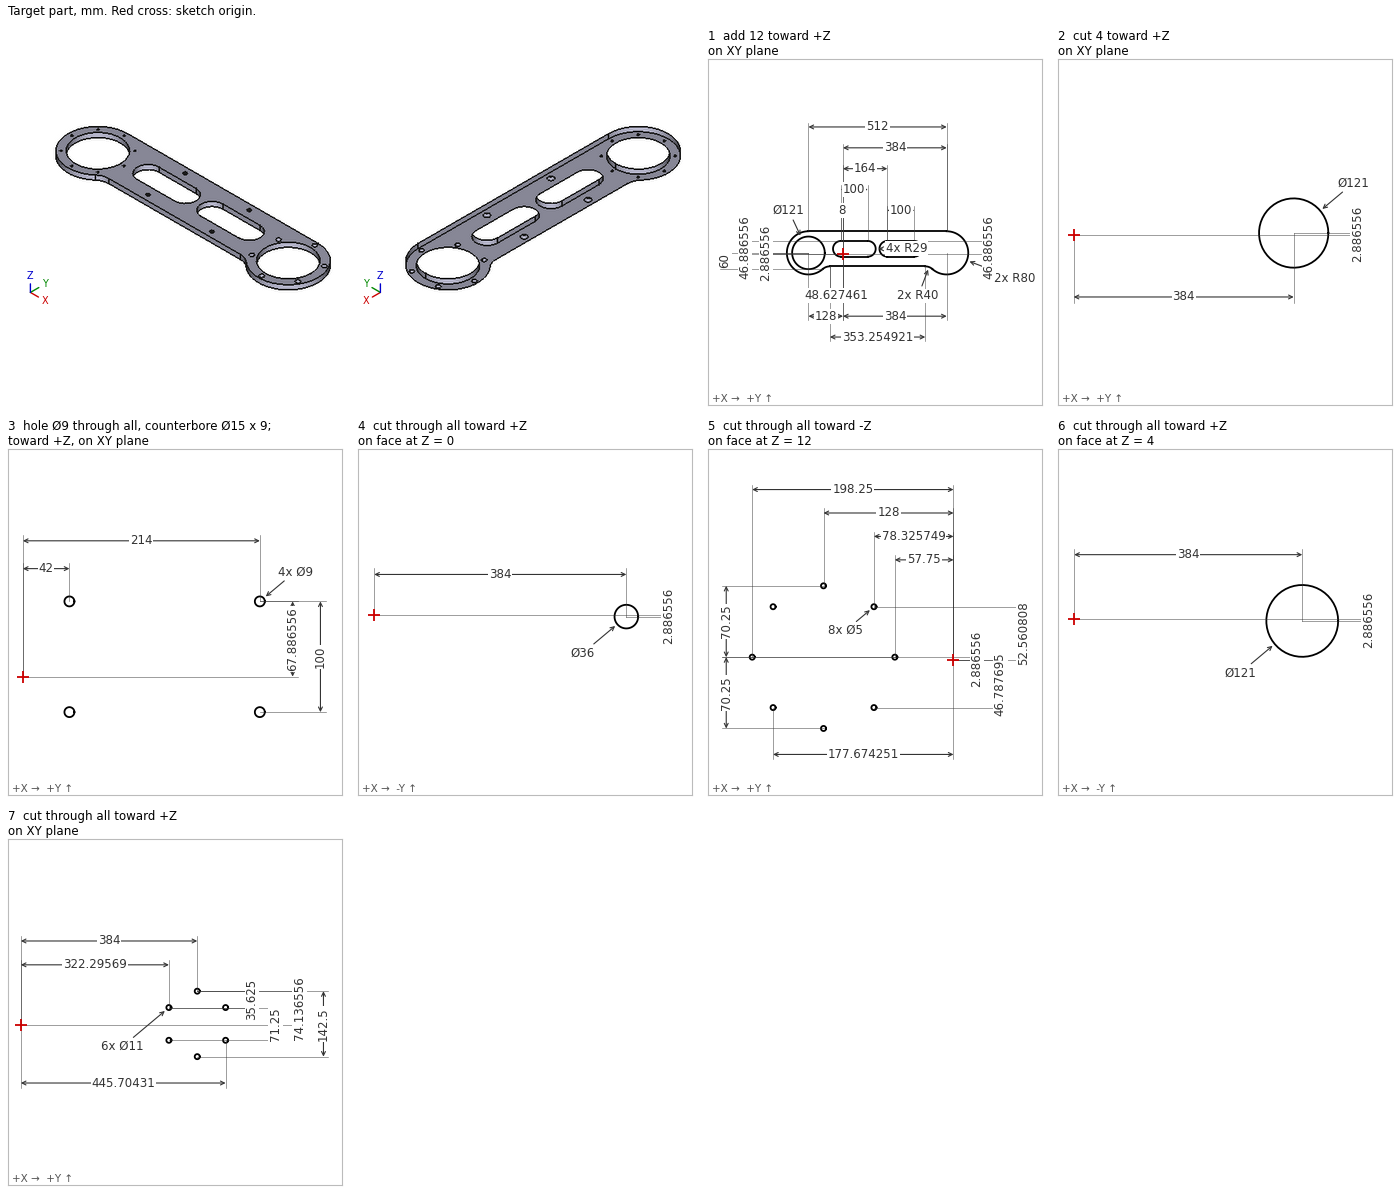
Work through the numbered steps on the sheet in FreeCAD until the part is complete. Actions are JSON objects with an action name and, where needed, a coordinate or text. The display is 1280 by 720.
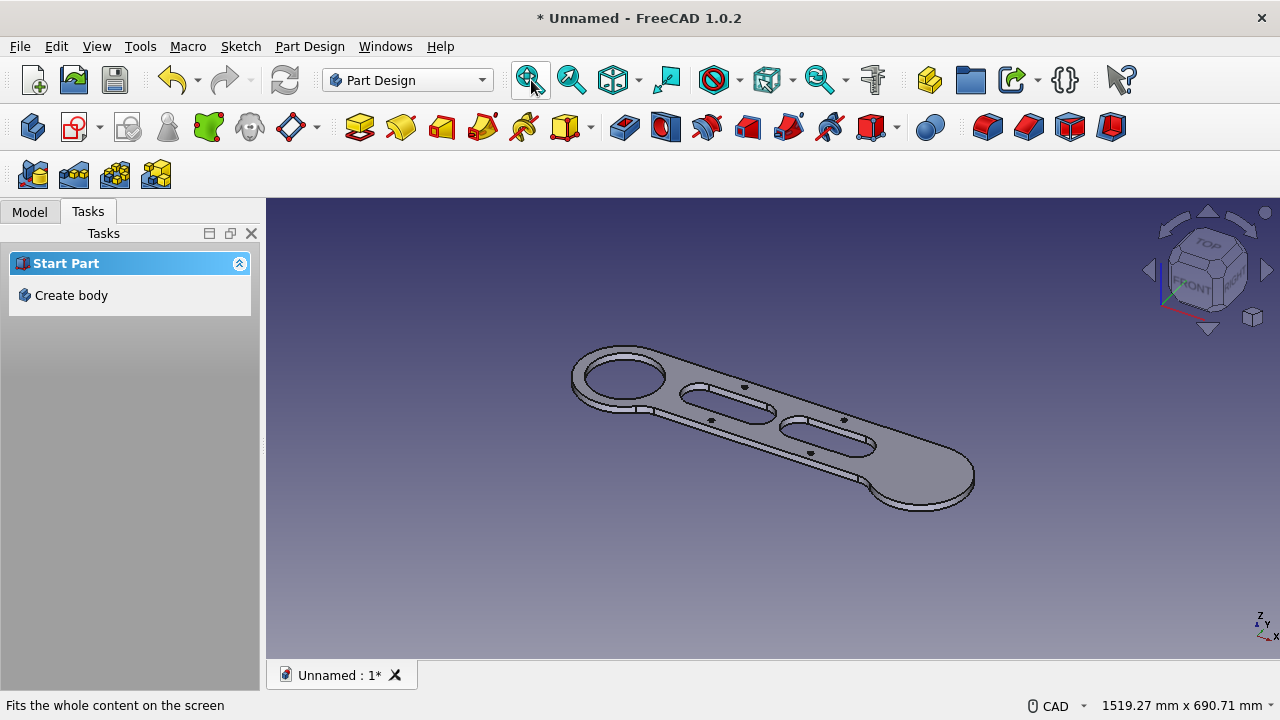
{"action": "key", "text": "5"}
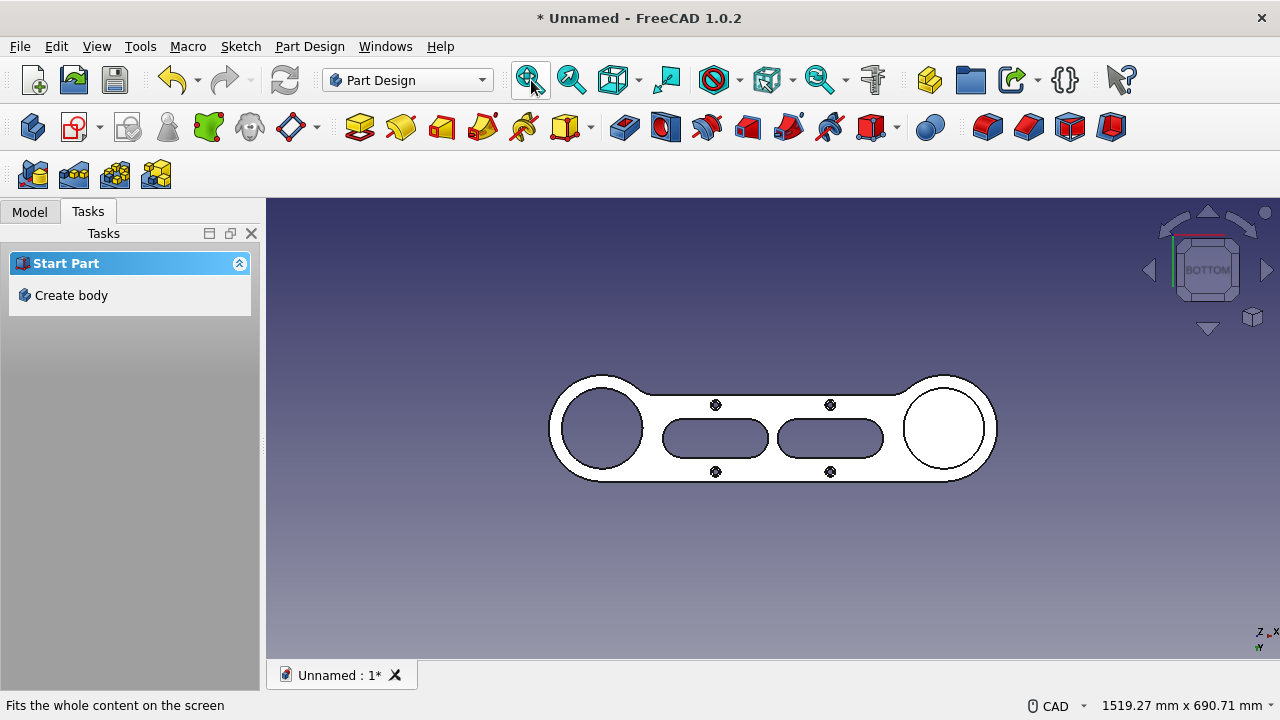
{"action": "left_click", "coordinate": [531, 80]}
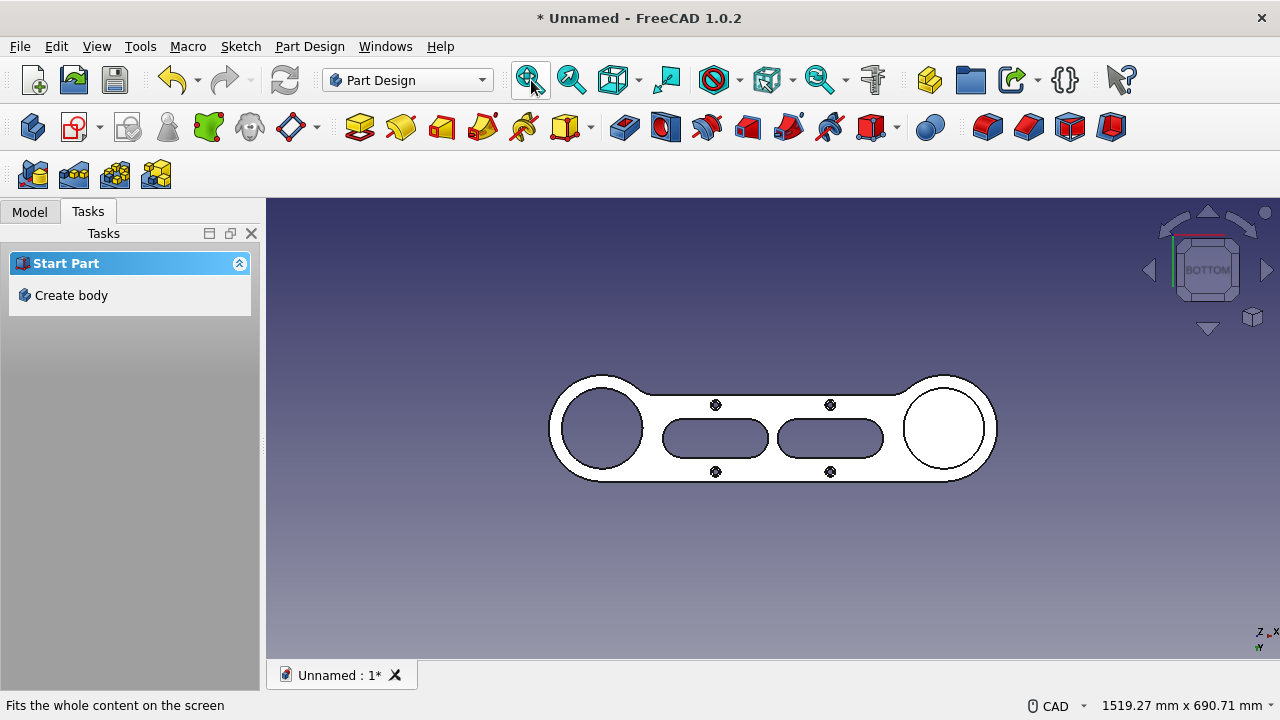
{"action": "left_click", "coordinate": [773, 412]}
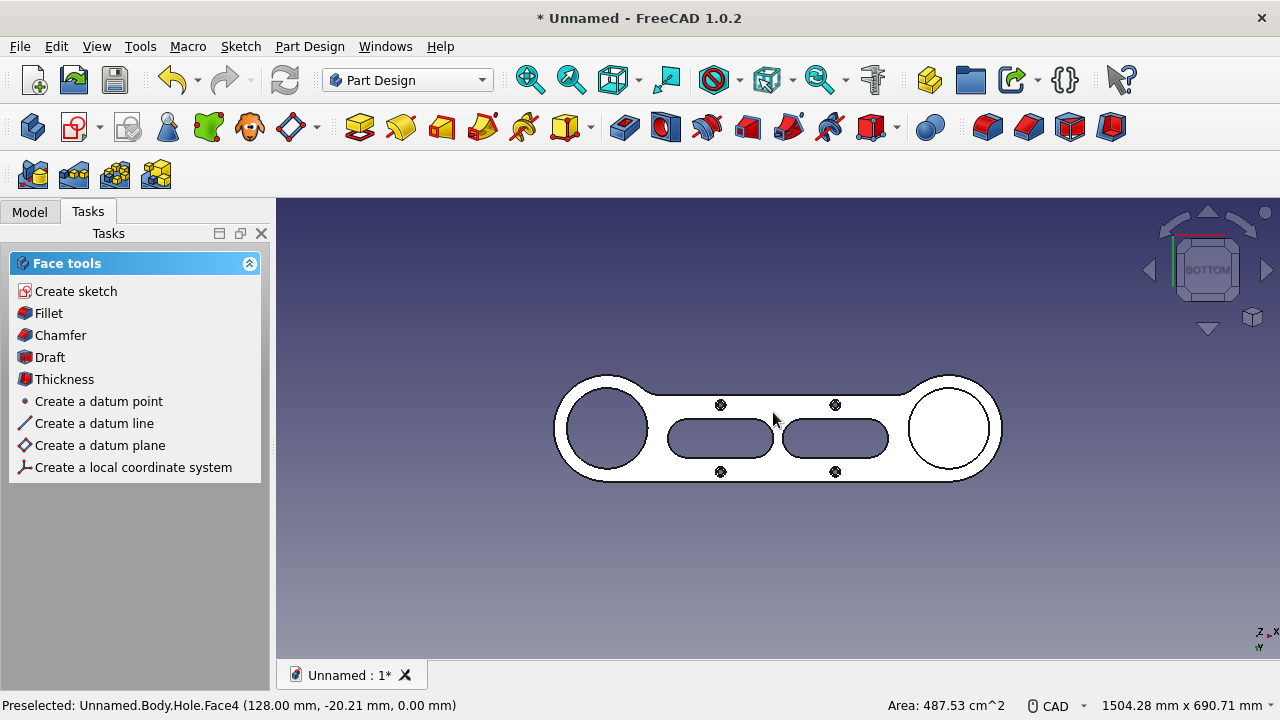
{"action": "left_click", "coordinate": [74, 128]}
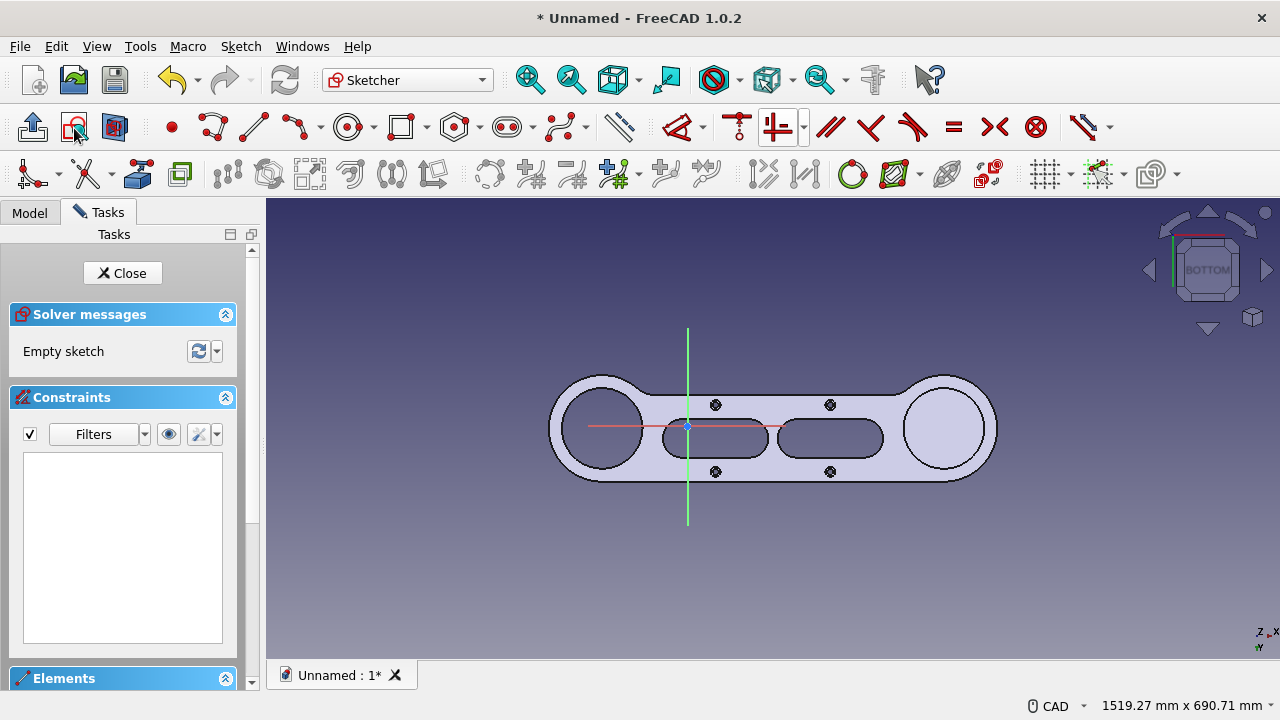
{"action": "scroll", "coordinate": [968, 428], "scroll_direction": "up", "scroll_amount": 12}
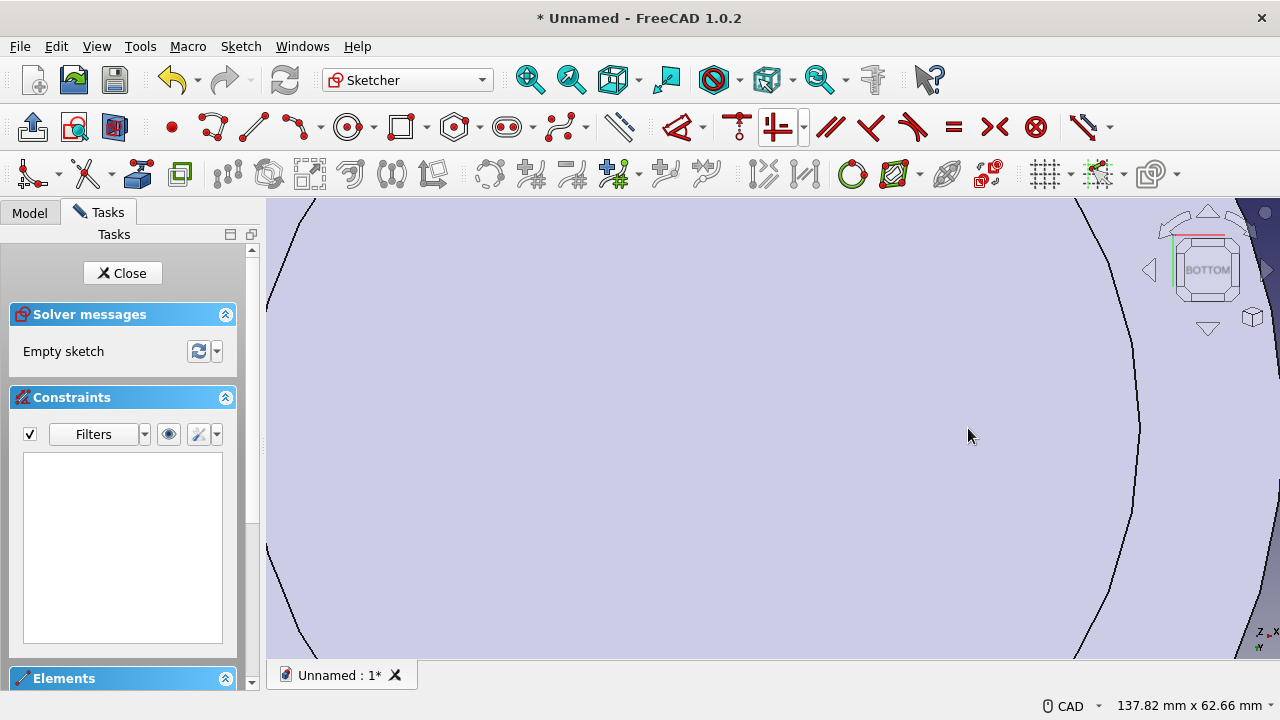
{"action": "left_click", "coordinate": [348, 128]}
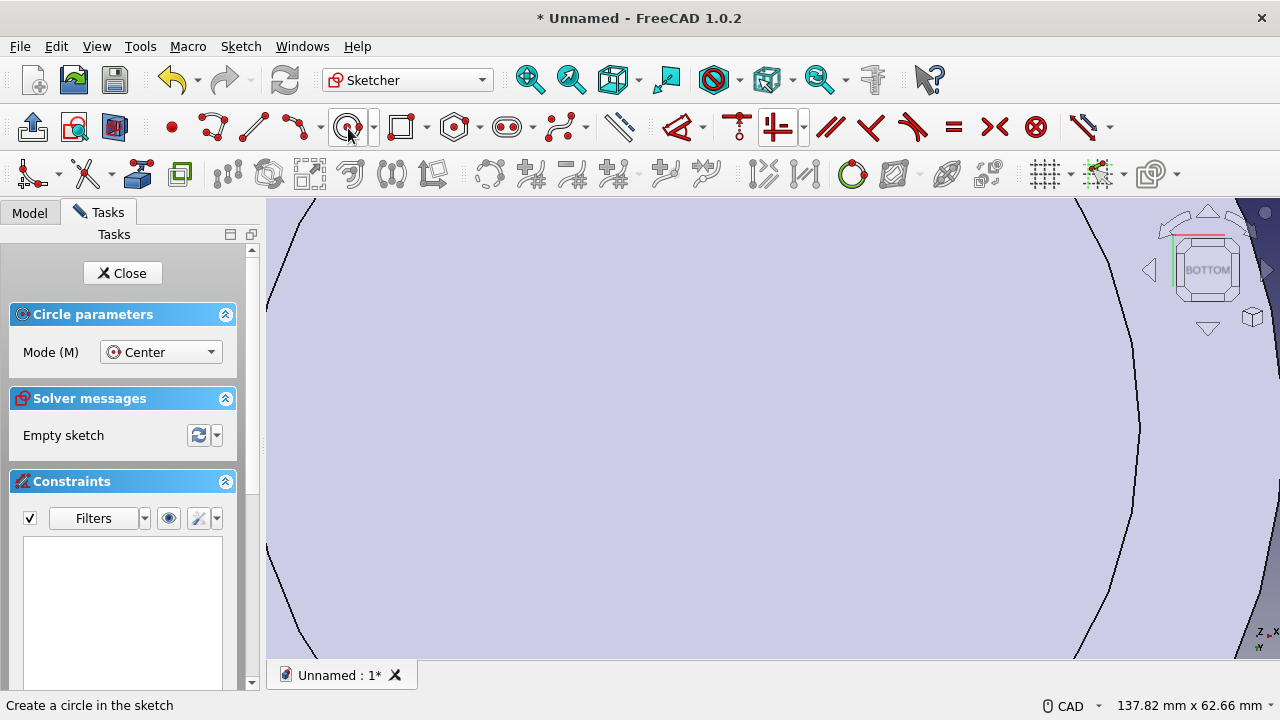
{"action": "left_click", "coordinate": [695, 428]}
{"action": "left_click", "coordinate": [789, 334]}
{"action": "key", "text": "Escape"}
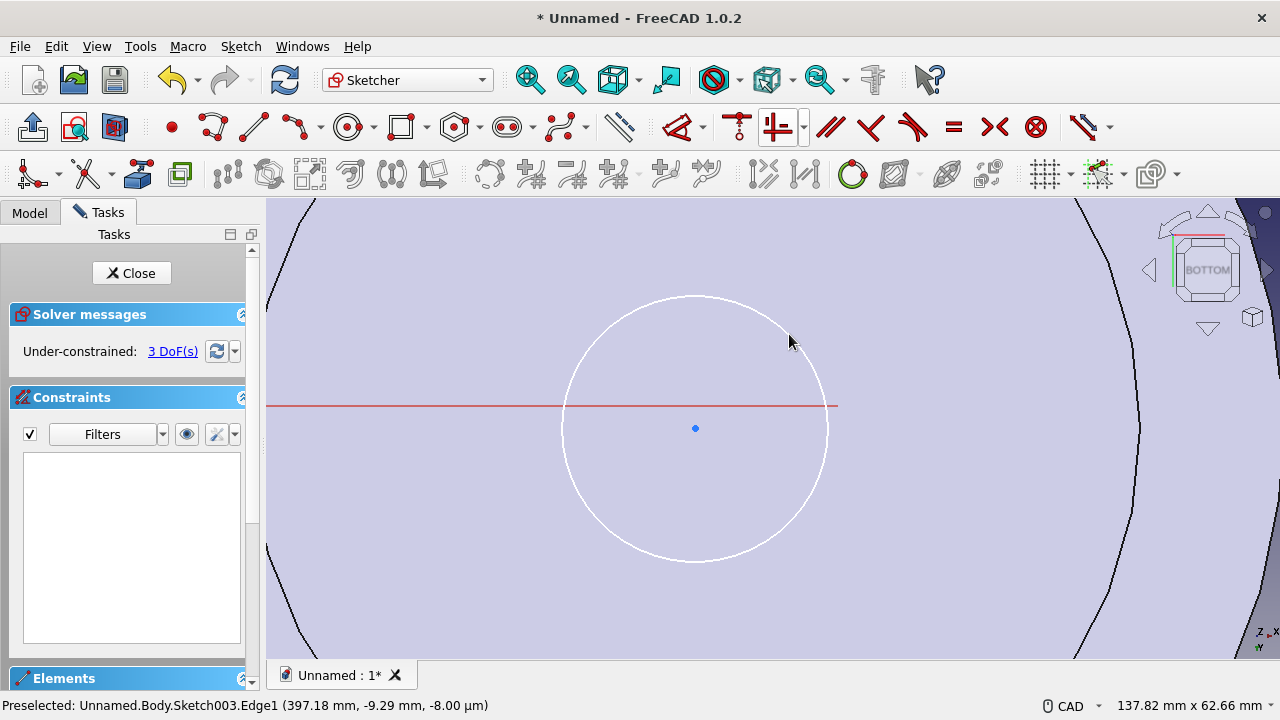
{"action": "left_click", "coordinate": [676, 128]}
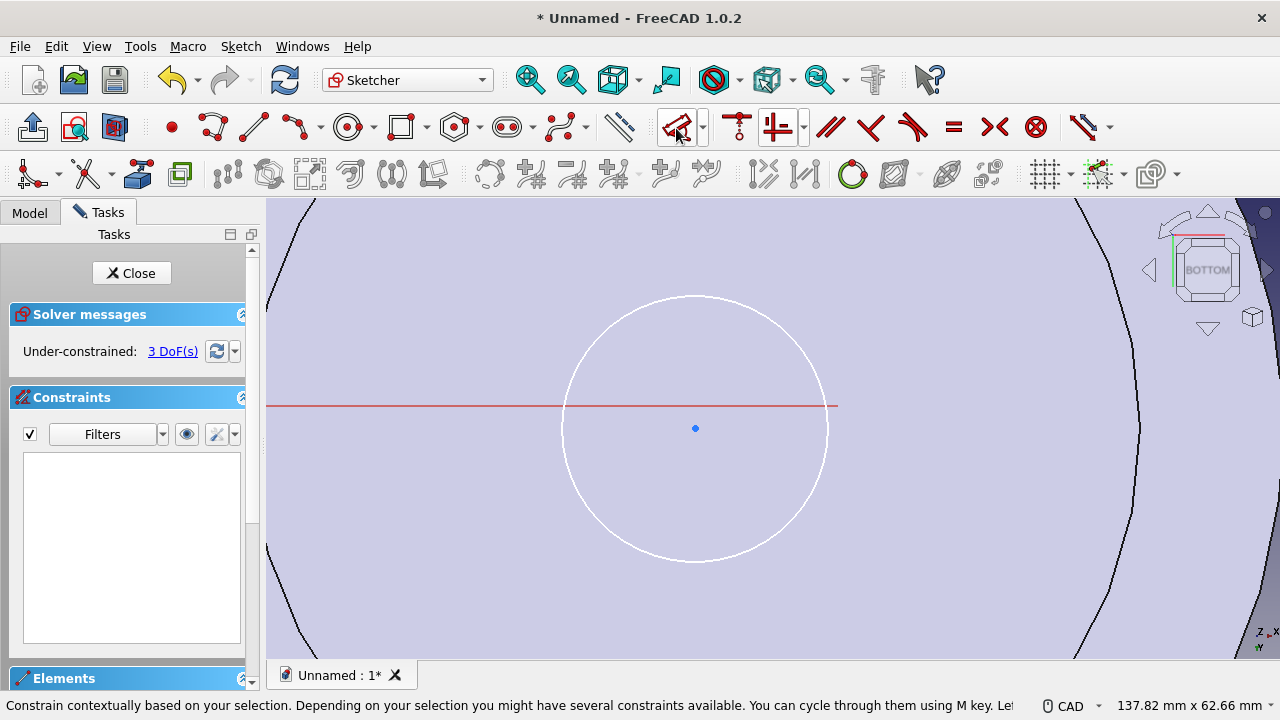
{"action": "left_click", "coordinate": [789, 335]}
{"action": "left_click", "coordinate": [812, 312]}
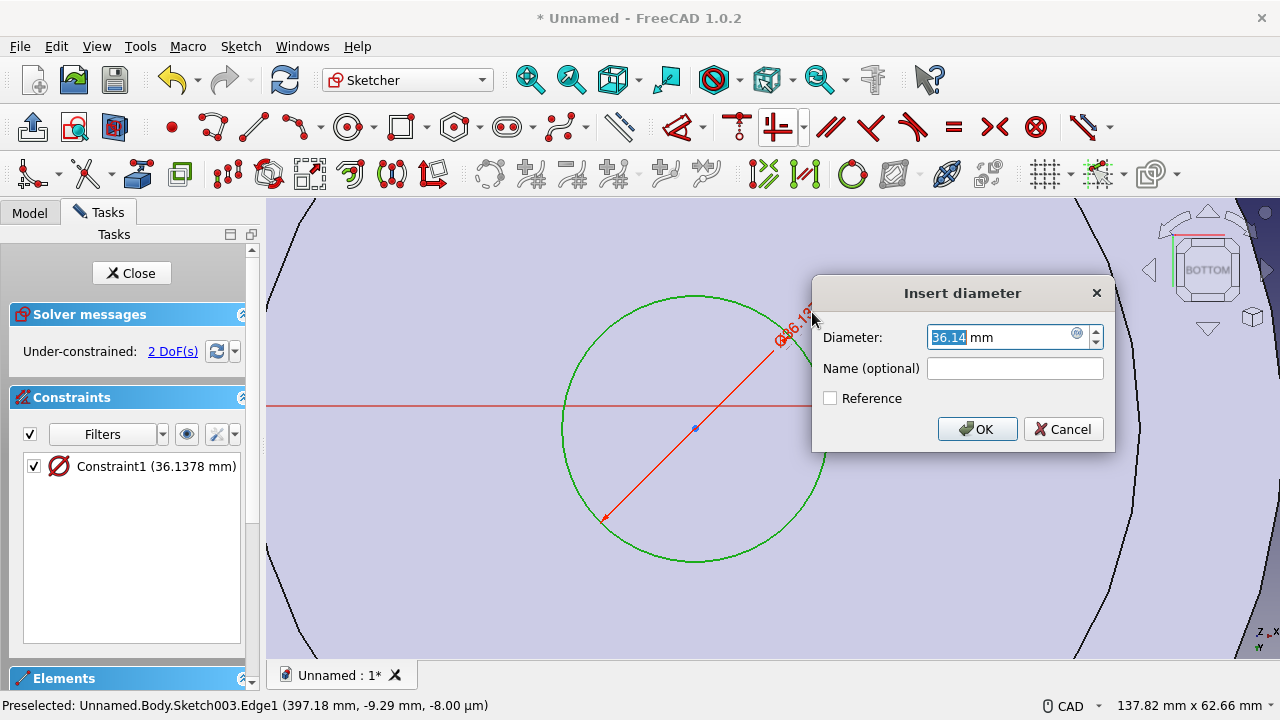
{"action": "type", "text": "36"}
{"action": "key", "text": "Return"}